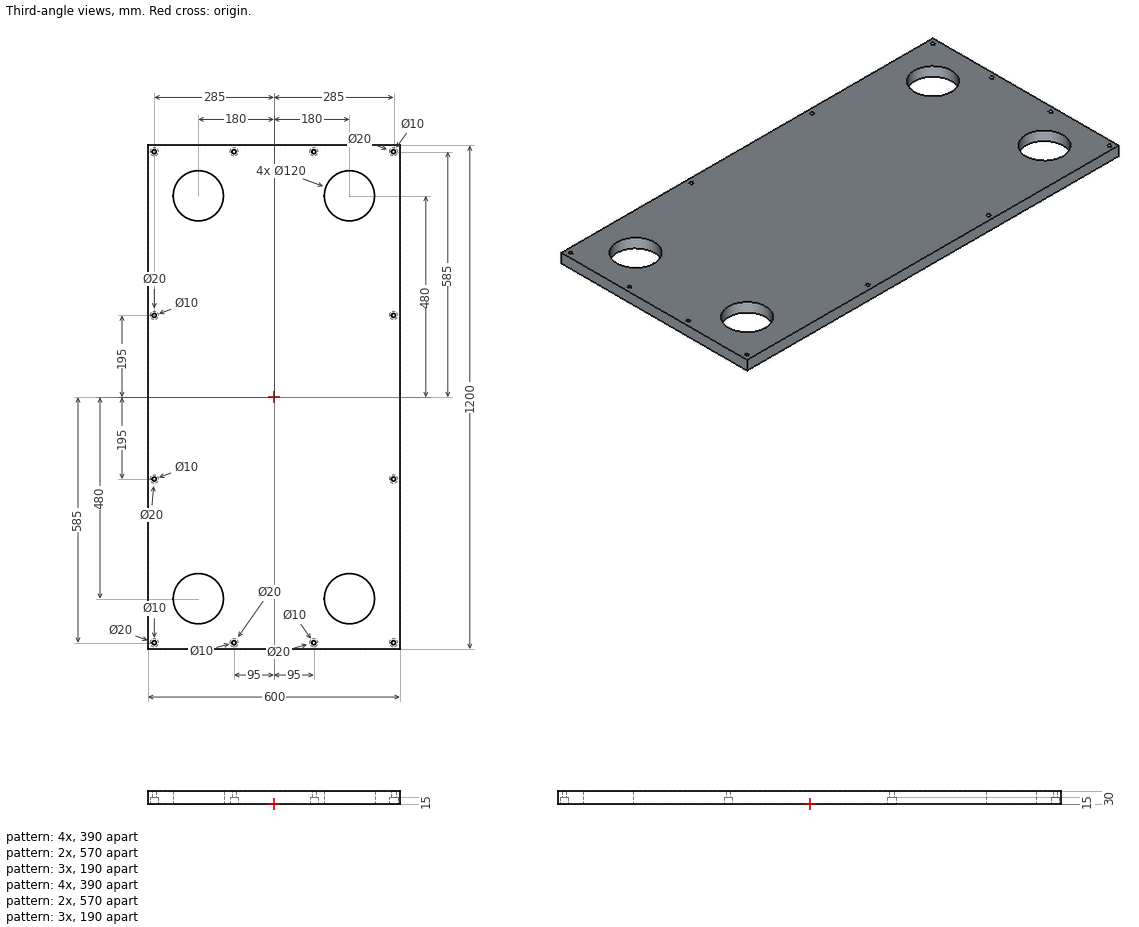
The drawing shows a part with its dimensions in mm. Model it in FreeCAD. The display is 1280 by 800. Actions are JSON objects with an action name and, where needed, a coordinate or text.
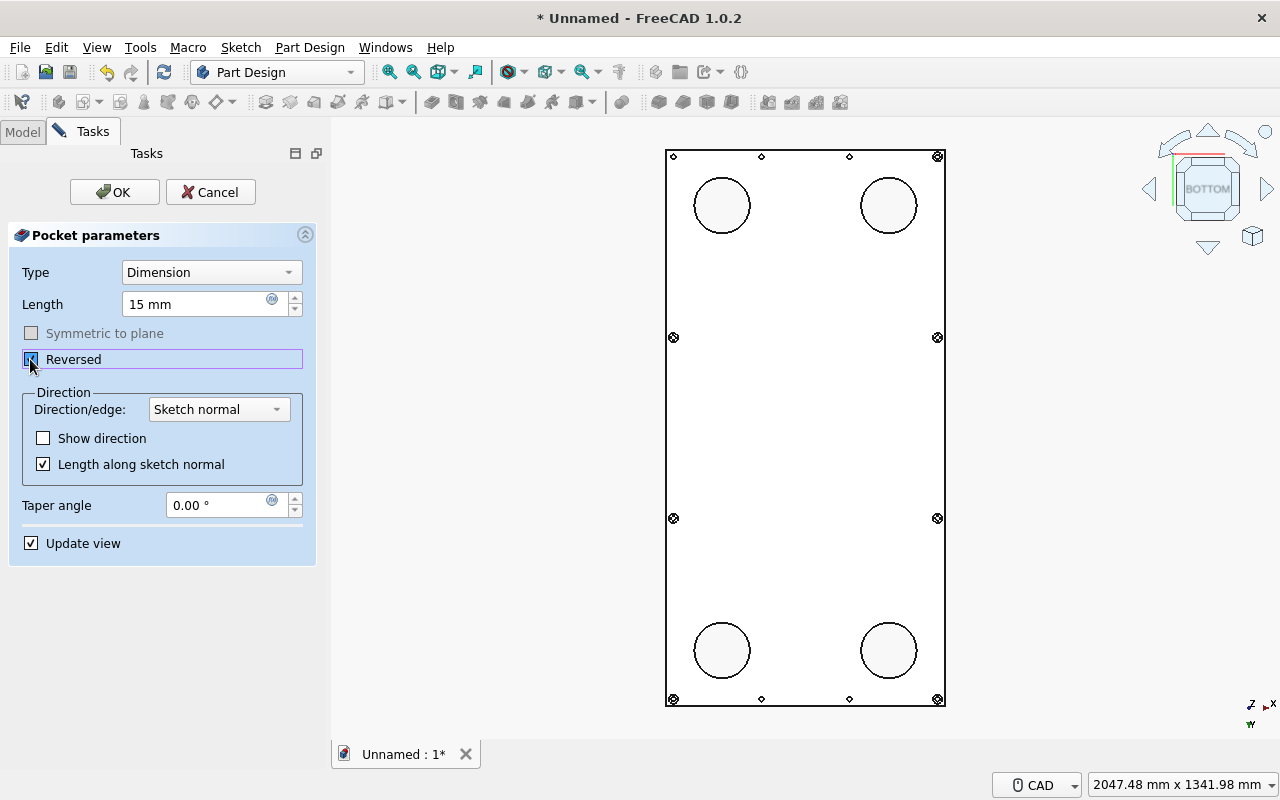
{"action": "left_click", "coordinate": [115, 192]}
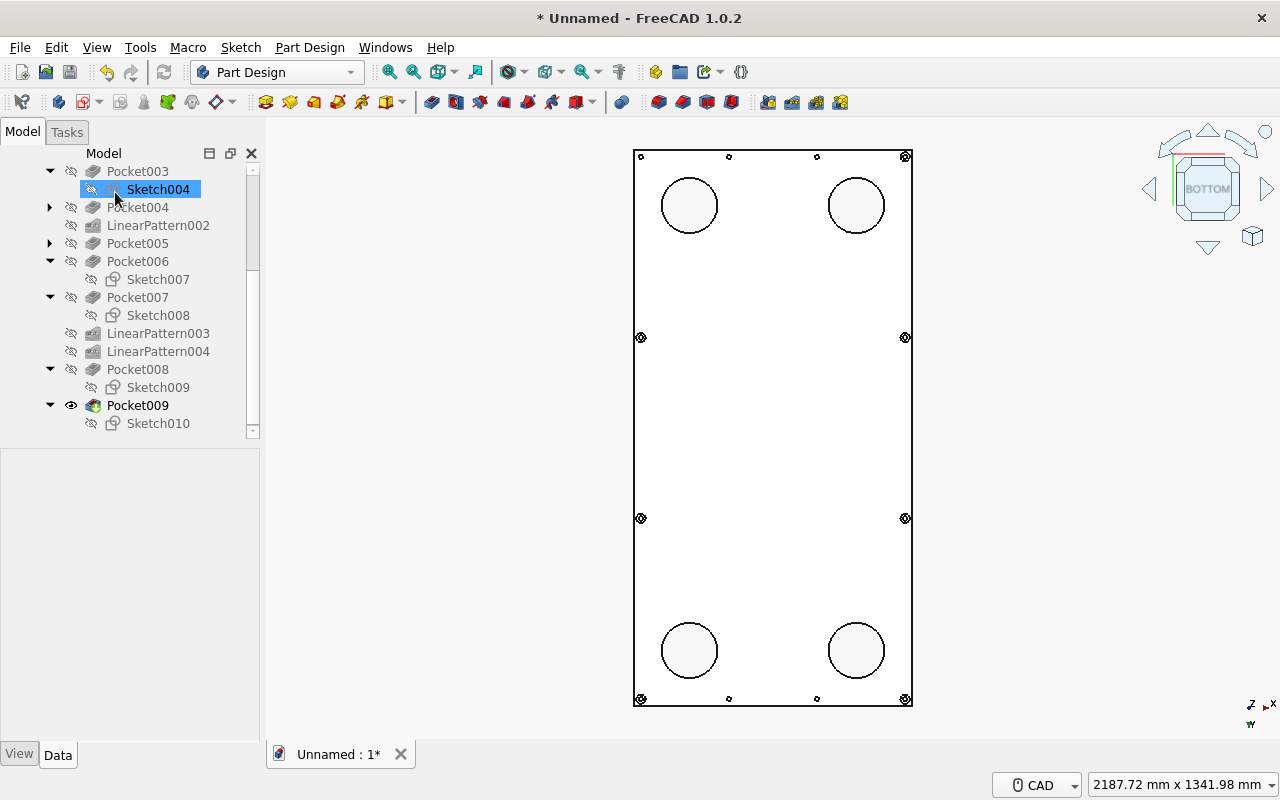
{"action": "left_click", "coordinate": [773, 427]}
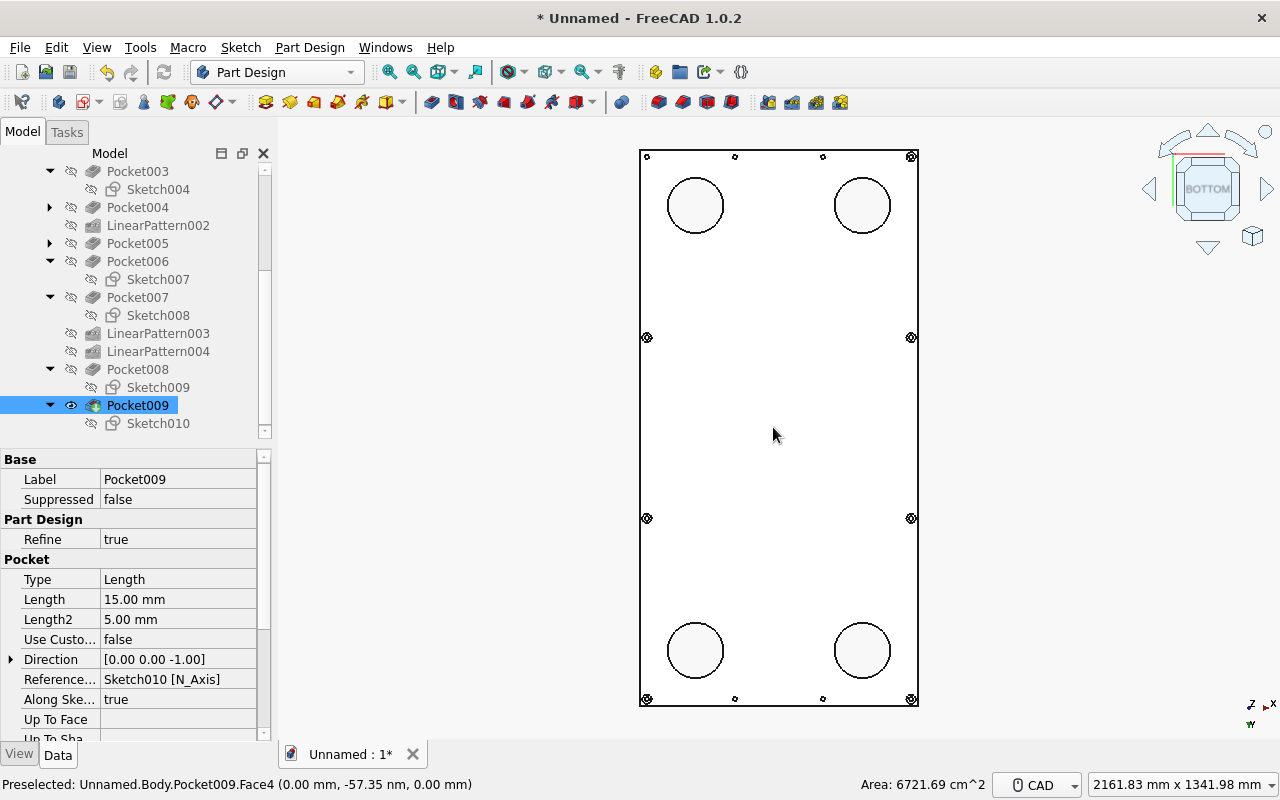
{"action": "left_click", "coordinate": [84, 102]}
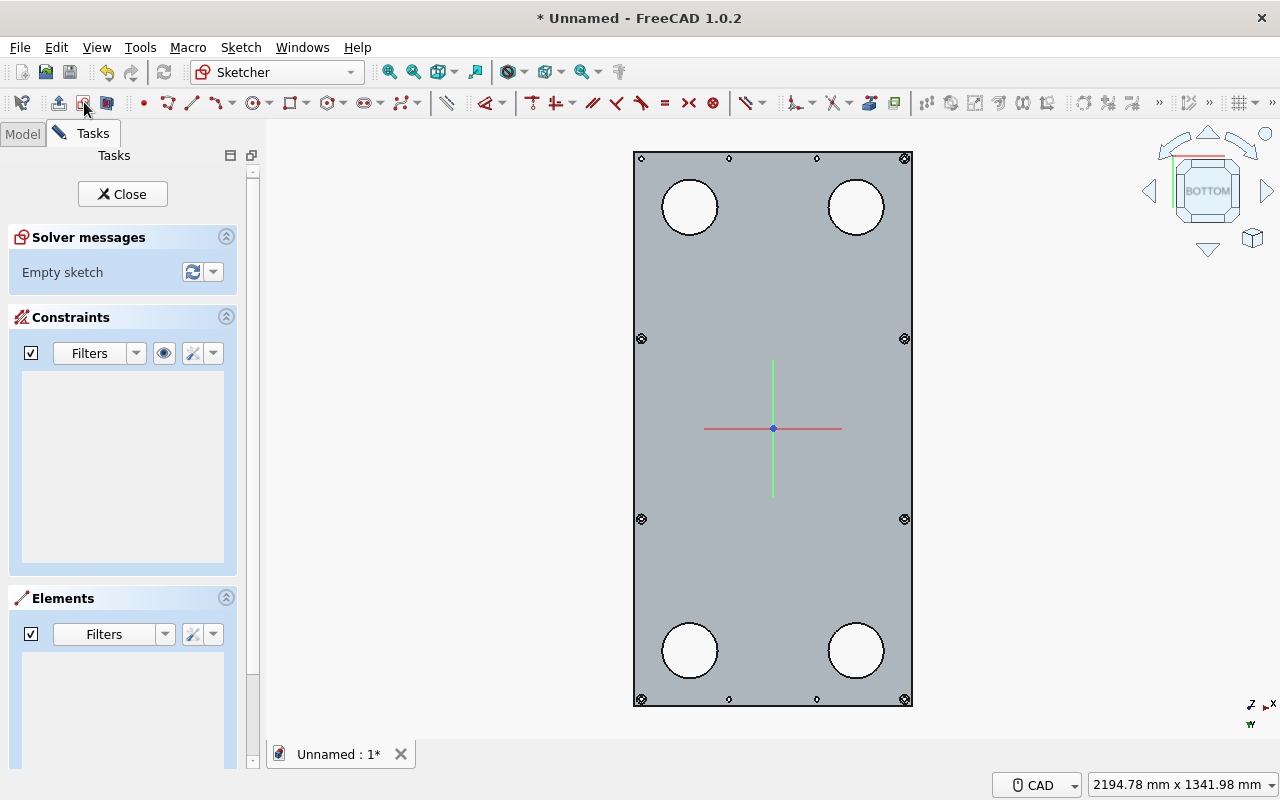
{"action": "scroll", "coordinate": [638, 147], "scroll_direction": "up", "scroll_amount": 15}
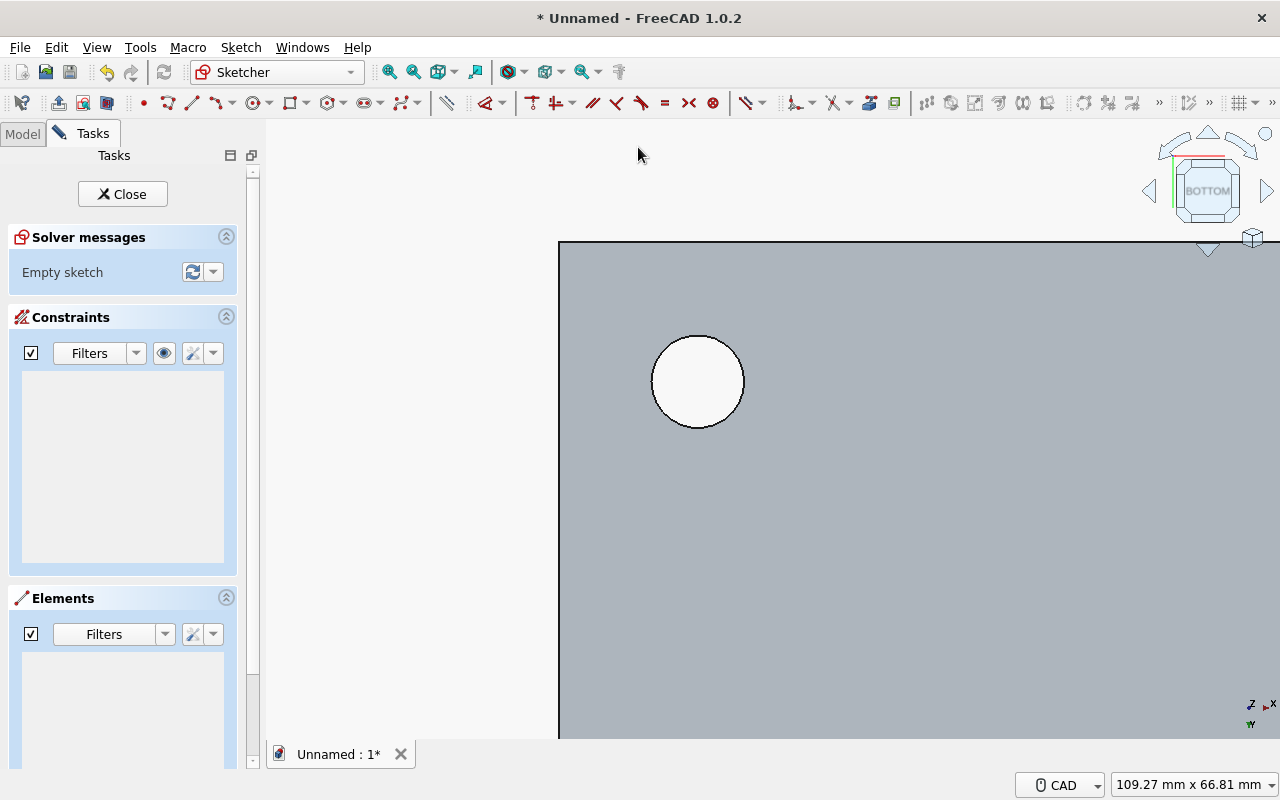
{"action": "scroll", "coordinate": [692, 343], "scroll_direction": "up", "scroll_amount": 4}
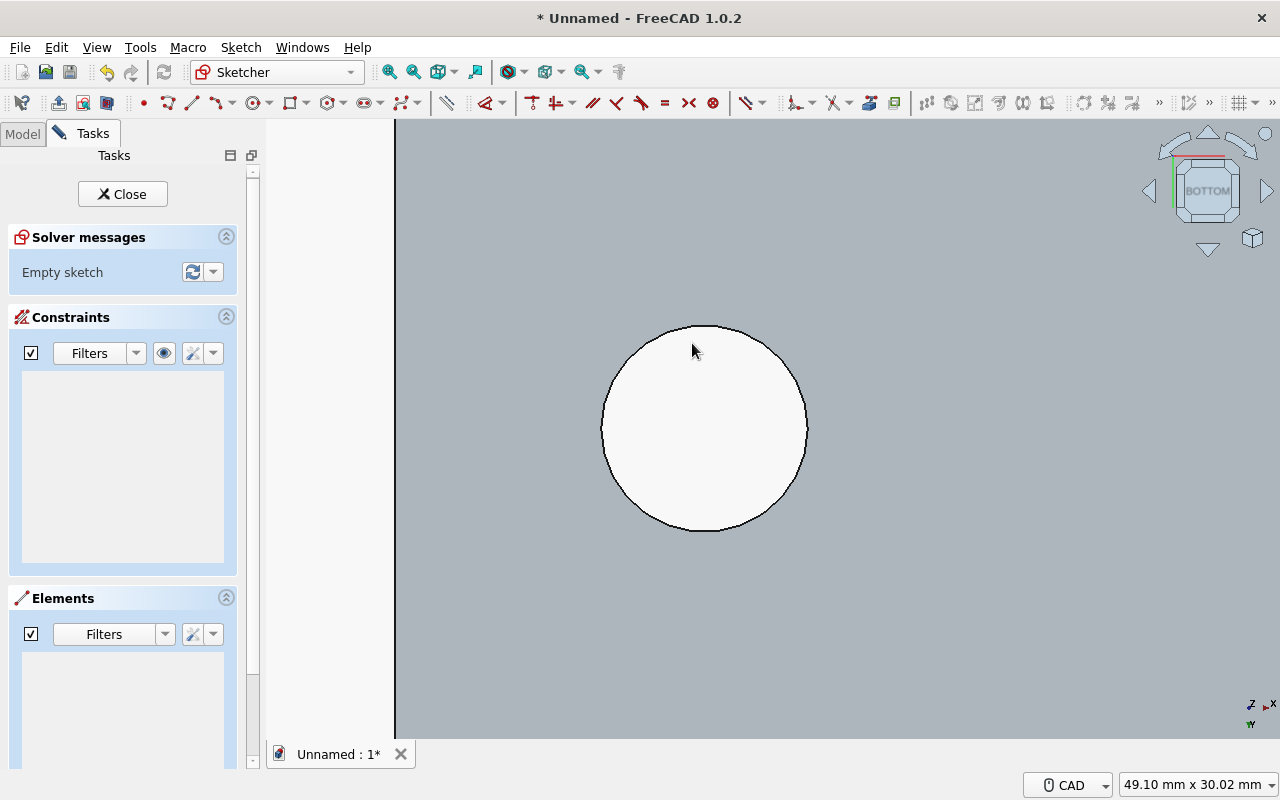
{"action": "left_click", "coordinate": [254, 104]}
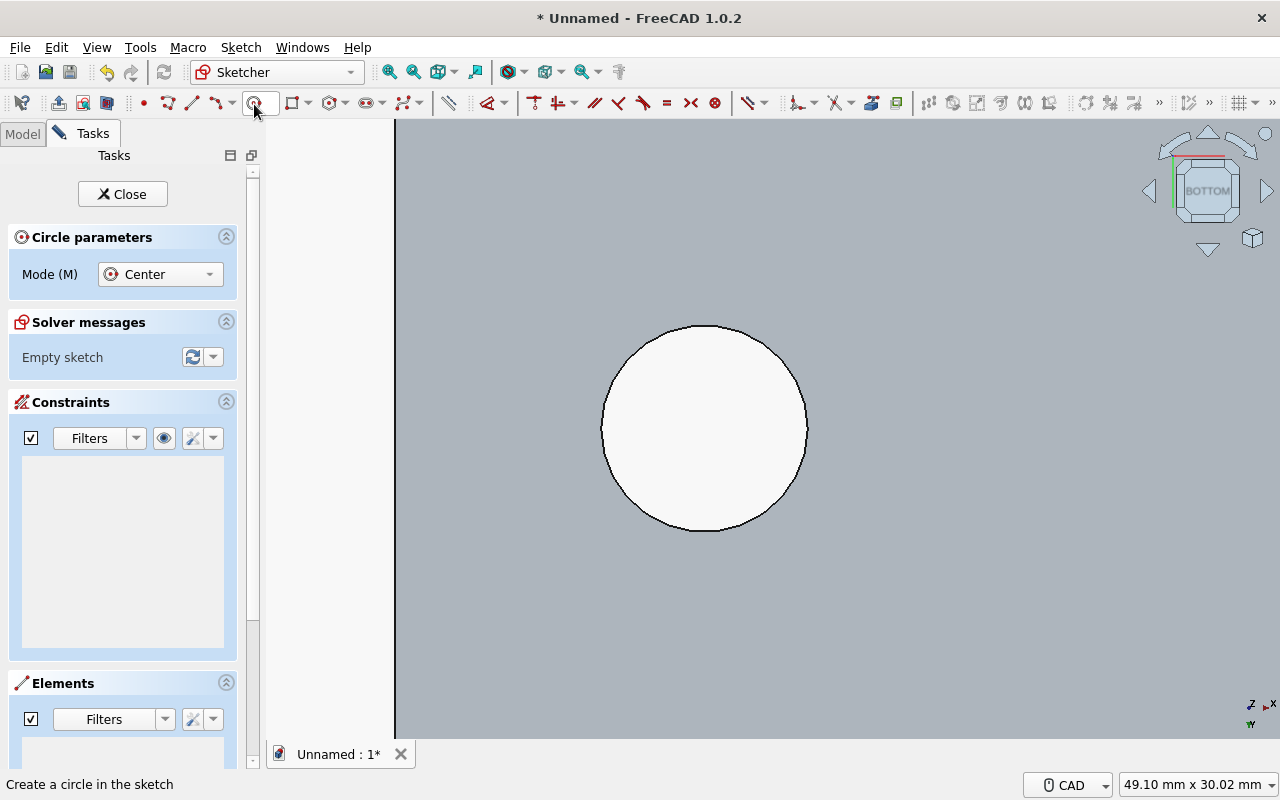
{"action": "left_click", "coordinate": [704, 429]}
{"action": "mouse_move", "coordinate": [851, 283]}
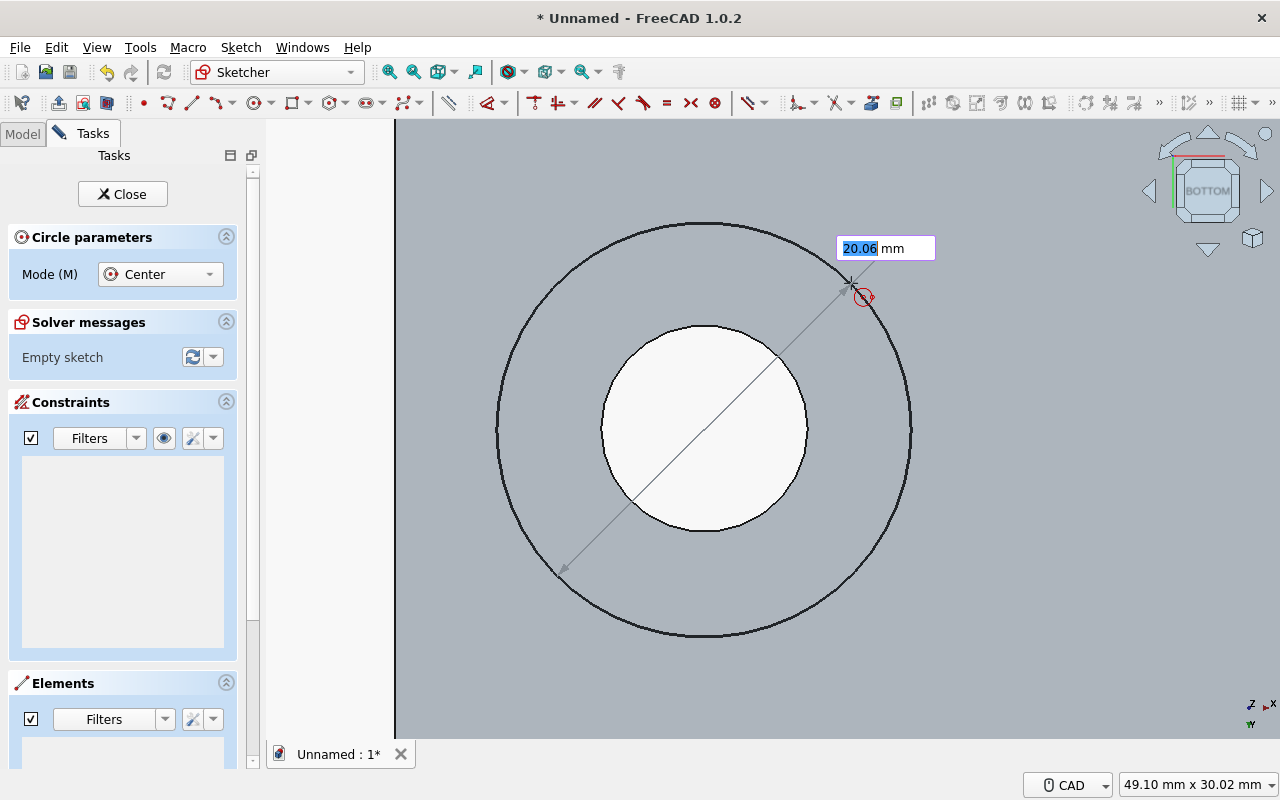
{"action": "type", "text": "20"}
{"action": "key", "text": "Return"}
{"action": "key", "text": "Escape"}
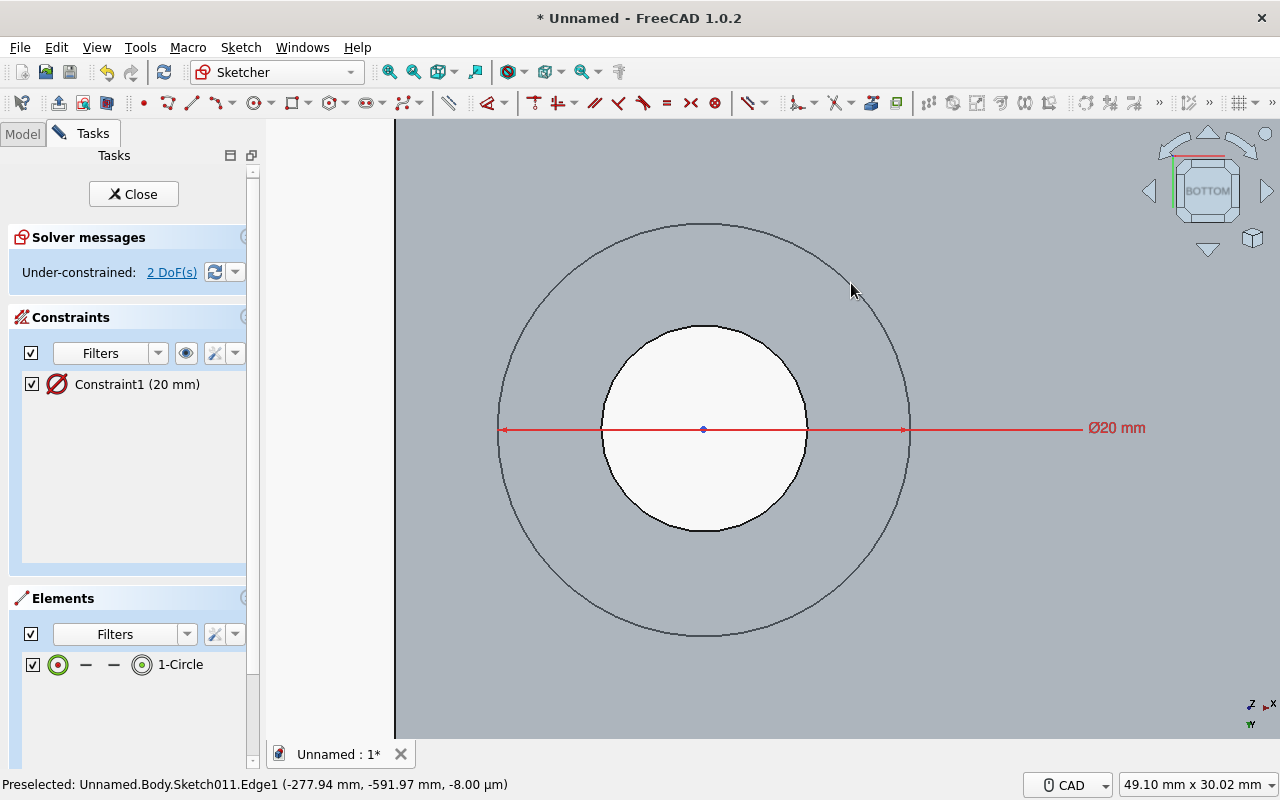
{"action": "key", "text": "d"}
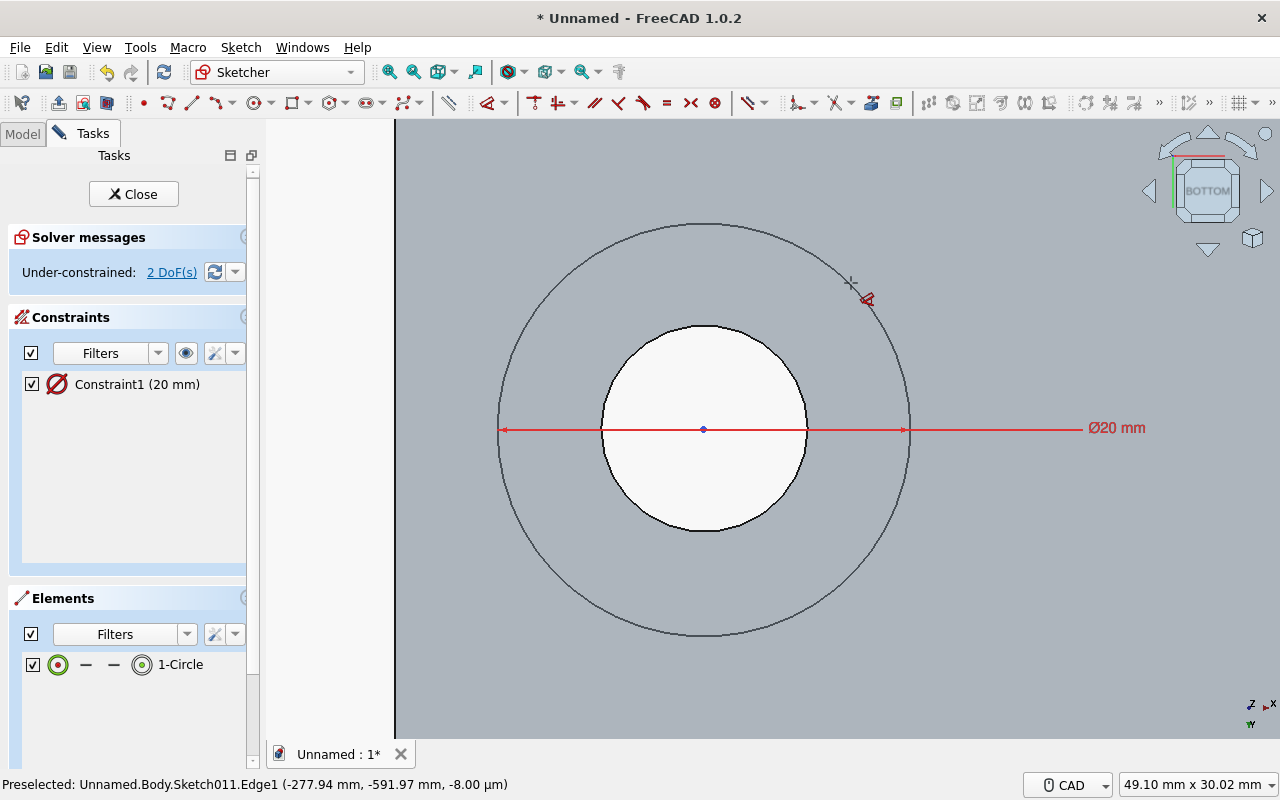
{"action": "left_click", "coordinate": [704, 430]}
{"action": "left_click", "coordinate": [815, 396]}